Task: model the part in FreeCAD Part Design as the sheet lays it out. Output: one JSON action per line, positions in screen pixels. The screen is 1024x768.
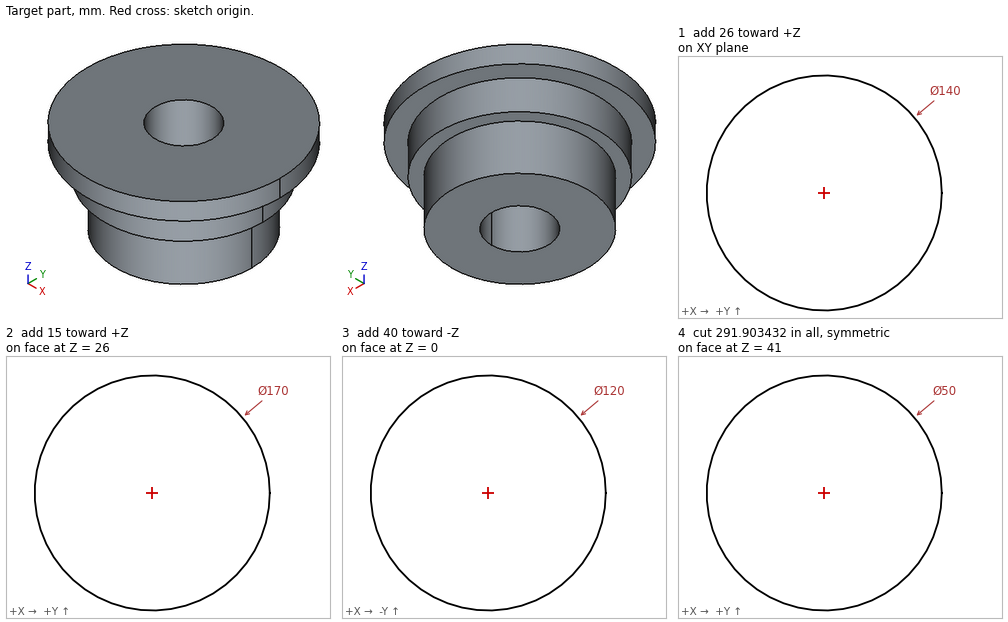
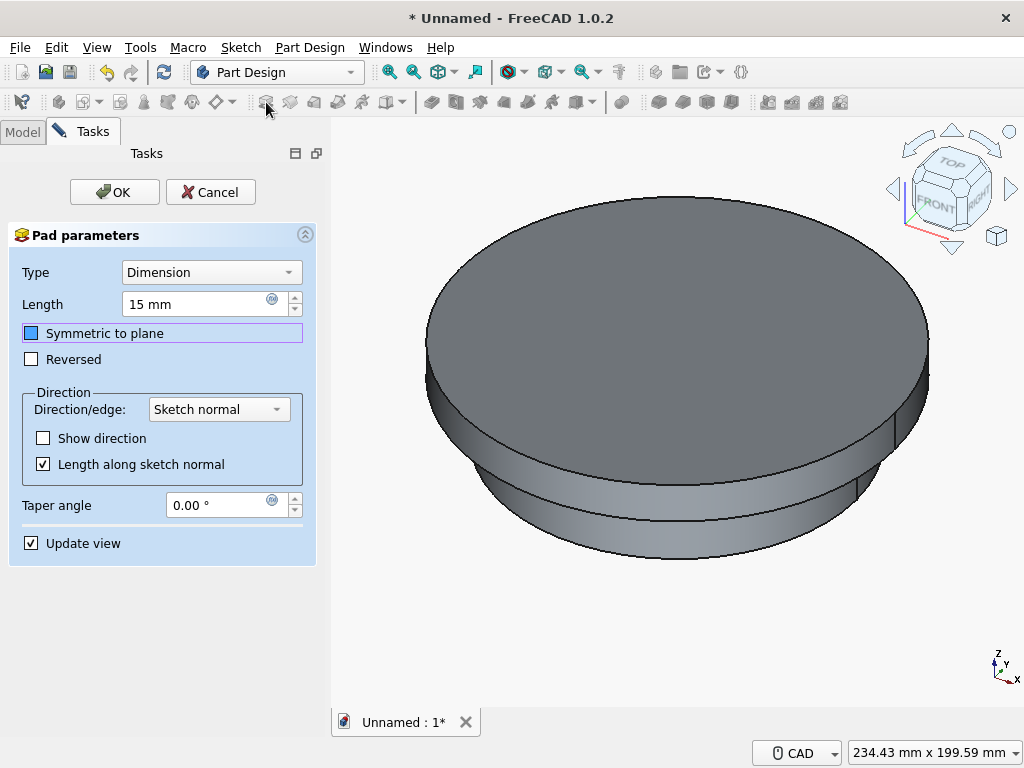
{"action": "left_click", "coordinate": [115, 192]}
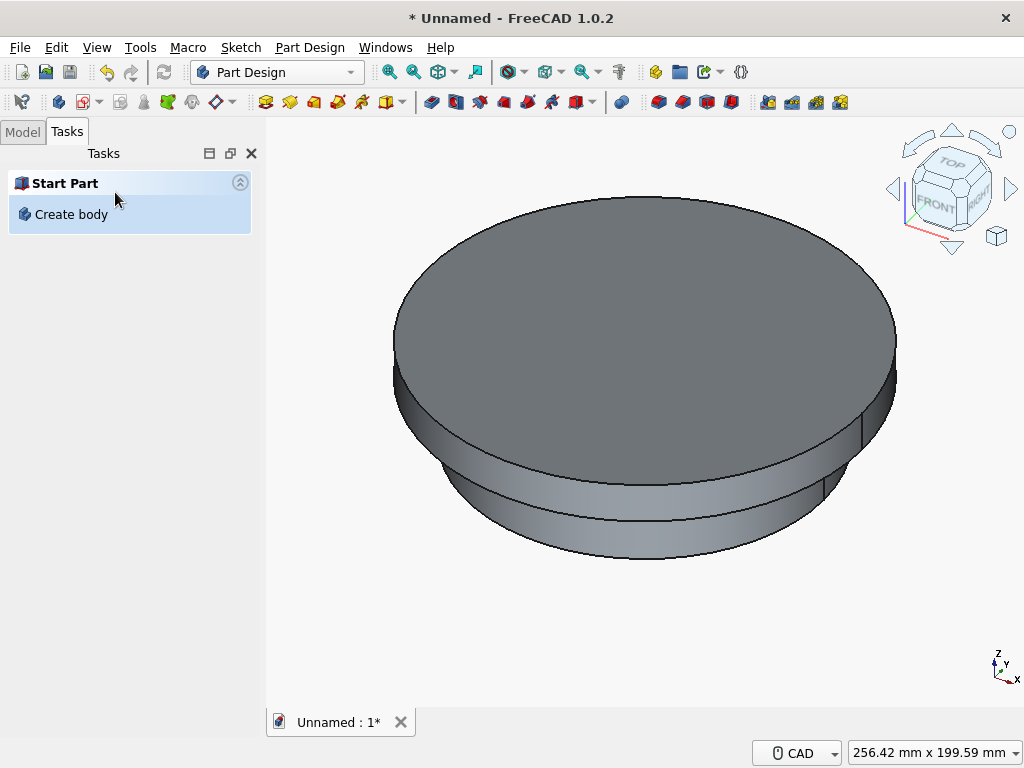
{"action": "key", "text": "5"}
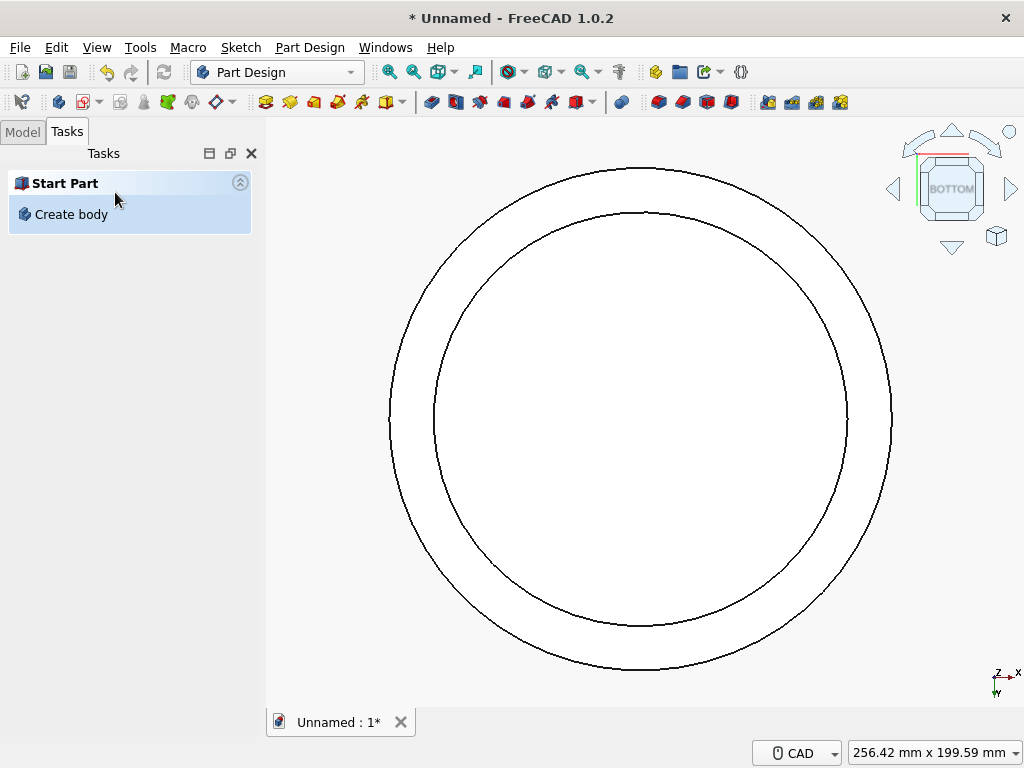
{"action": "left_click", "coordinate": [641, 418]}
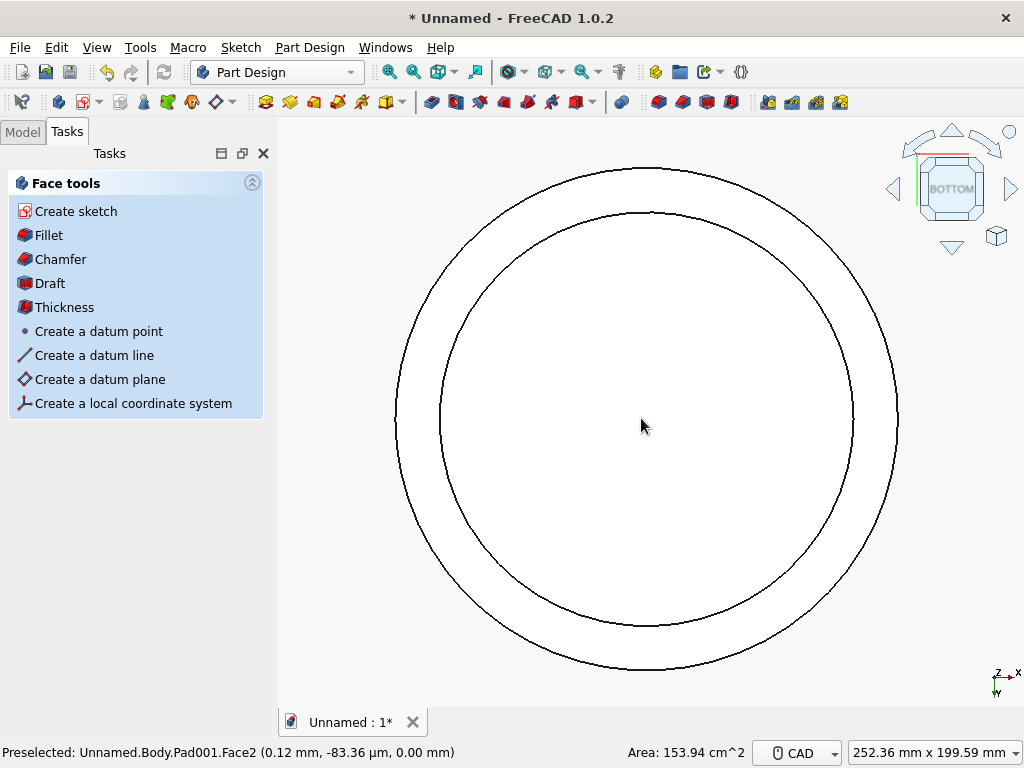
{"action": "left_click", "coordinate": [84, 102]}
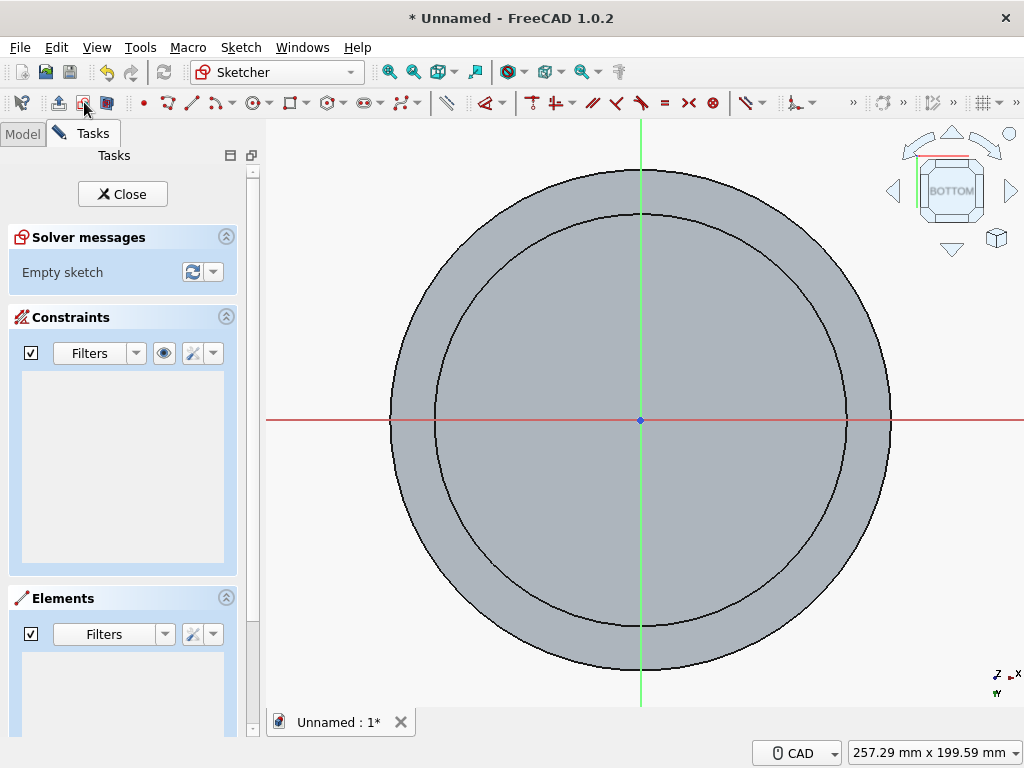
{"action": "key", "text": "g c"}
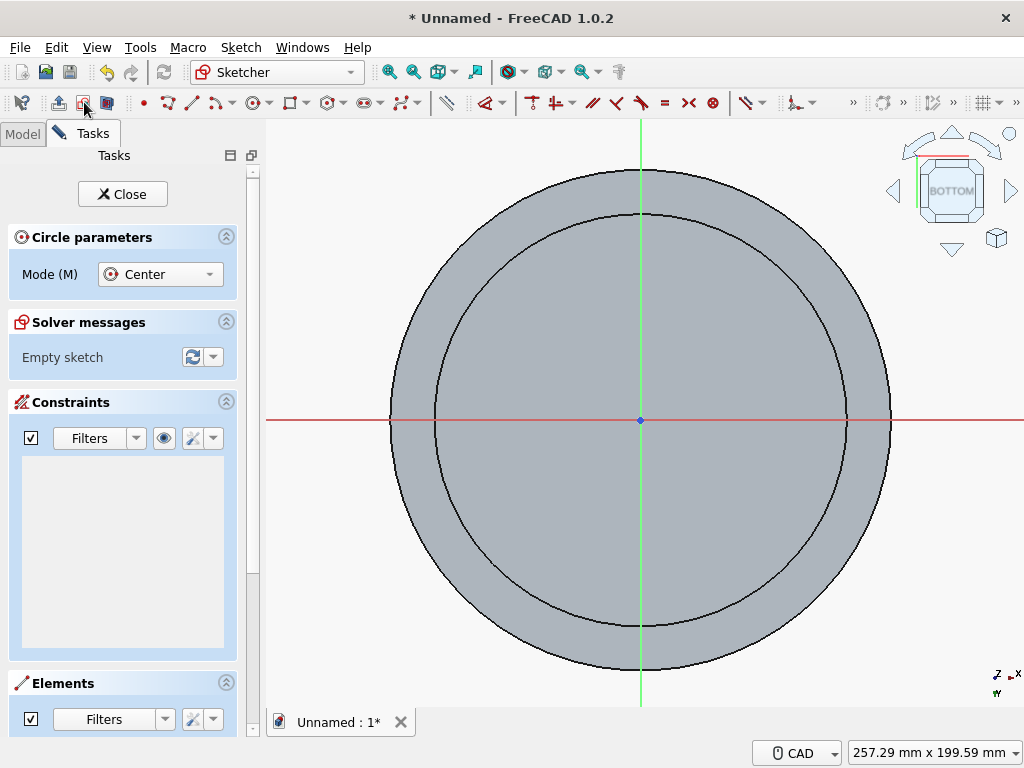
{"action": "left_click", "coordinate": [641, 420]}
{"action": "left_click", "coordinate": [766, 295]}
{"action": "key", "text": "Escape"}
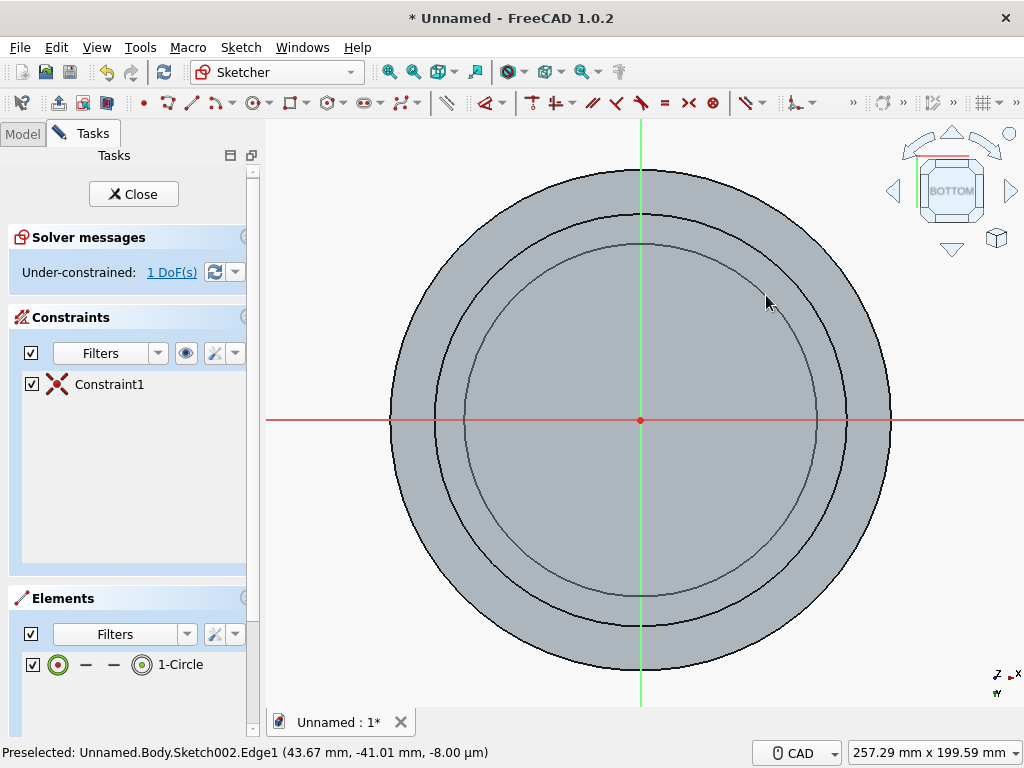
{"action": "key", "text": "d"}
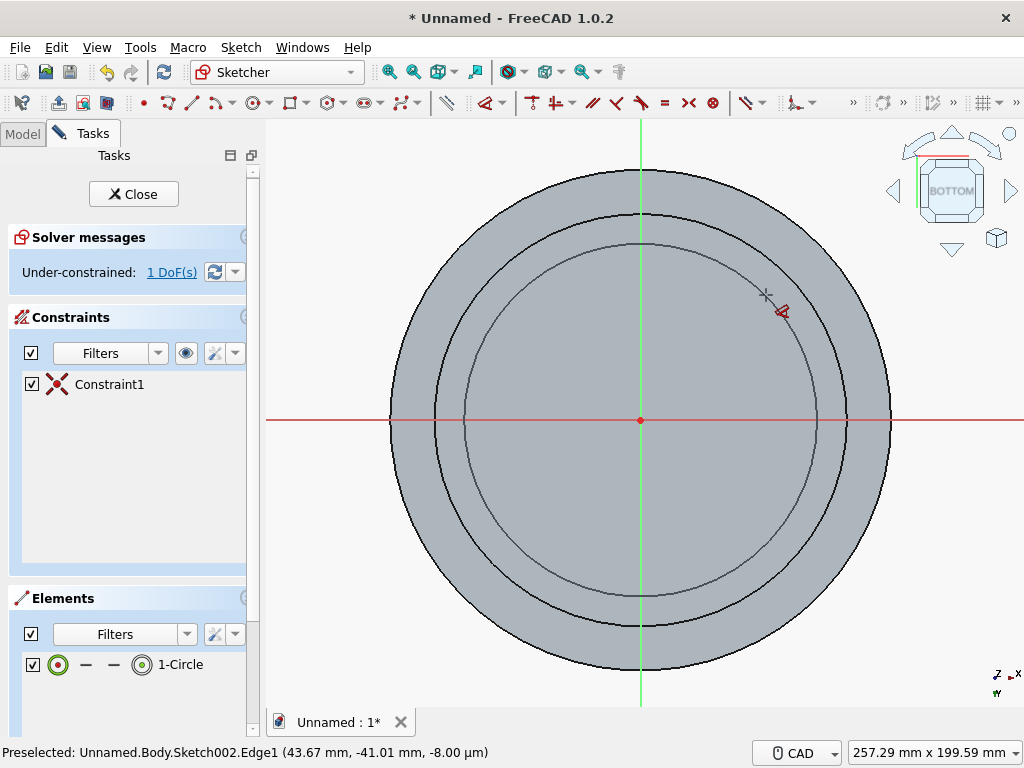
{"action": "left_click", "coordinate": [765, 295]}
{"action": "left_click", "coordinate": [788, 272]}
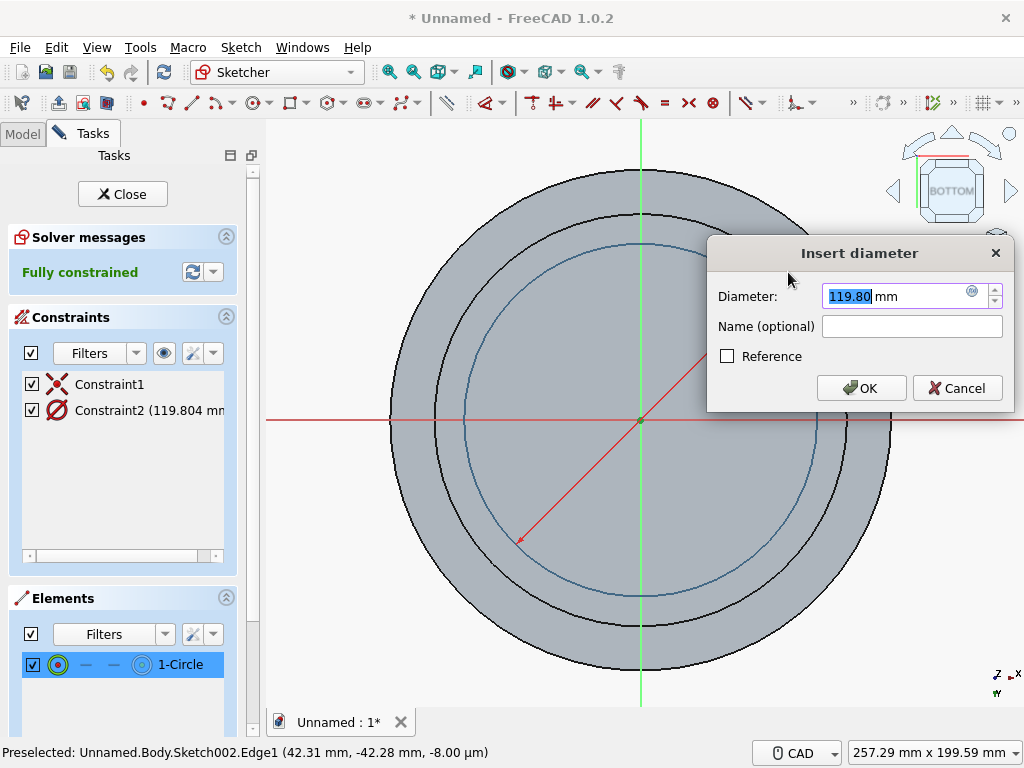
{"action": "type", "text": "120"}
{"action": "key", "text": "Return"}
{"action": "key", "text": "Escape"}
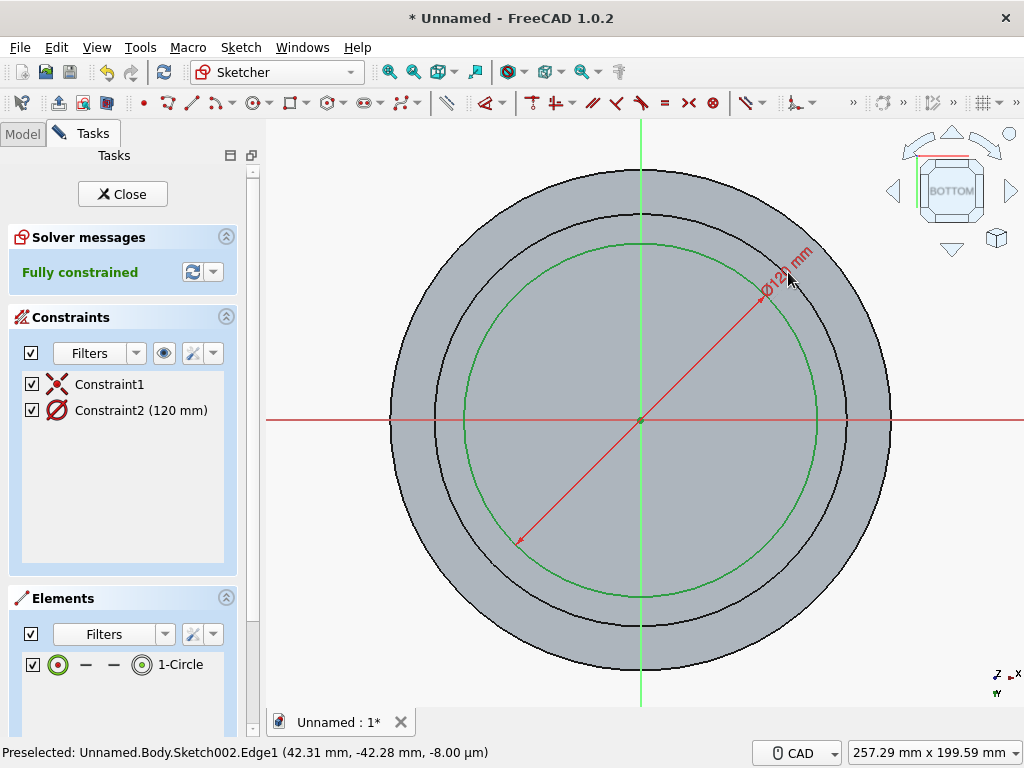
{"action": "left_click", "coordinate": [123, 194]}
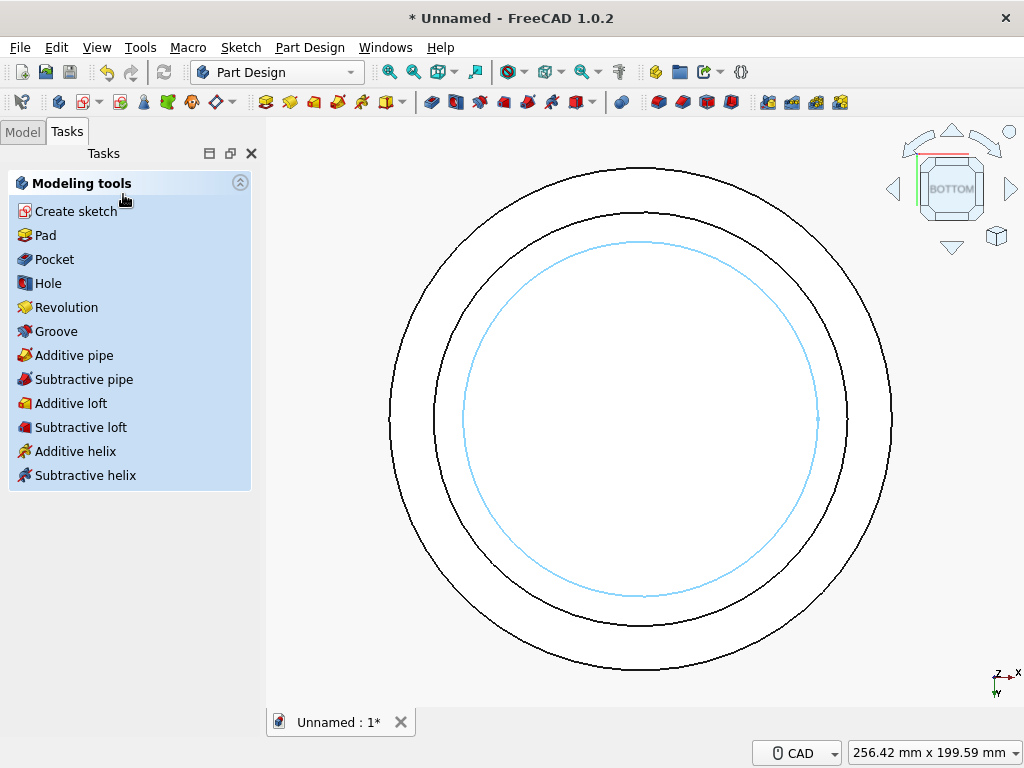
{"action": "left_click", "coordinate": [266, 102]}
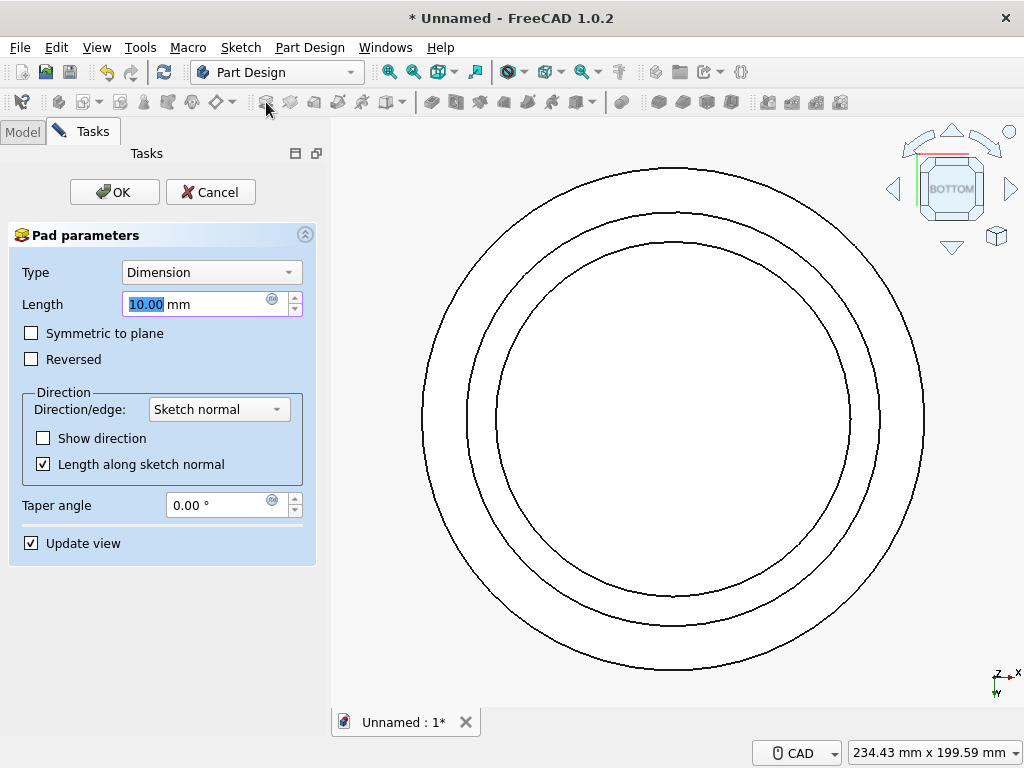
{"action": "type", "text": "40"}
{"action": "key", "text": "Tab"}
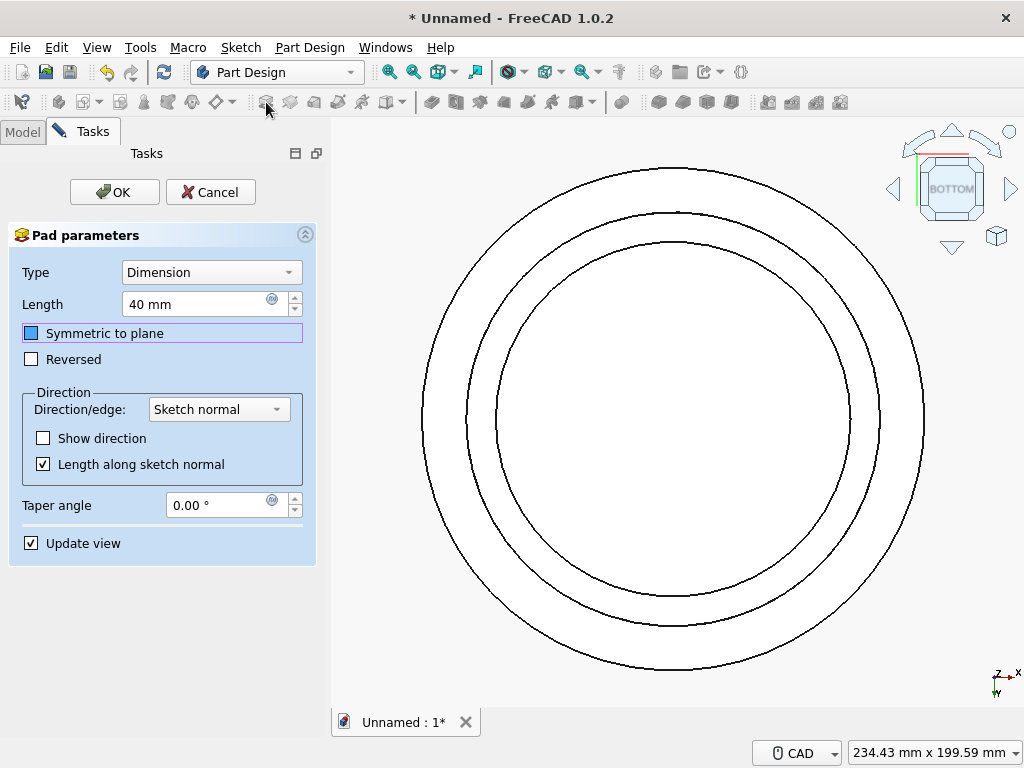
{"action": "left_click", "coordinate": [115, 192]}